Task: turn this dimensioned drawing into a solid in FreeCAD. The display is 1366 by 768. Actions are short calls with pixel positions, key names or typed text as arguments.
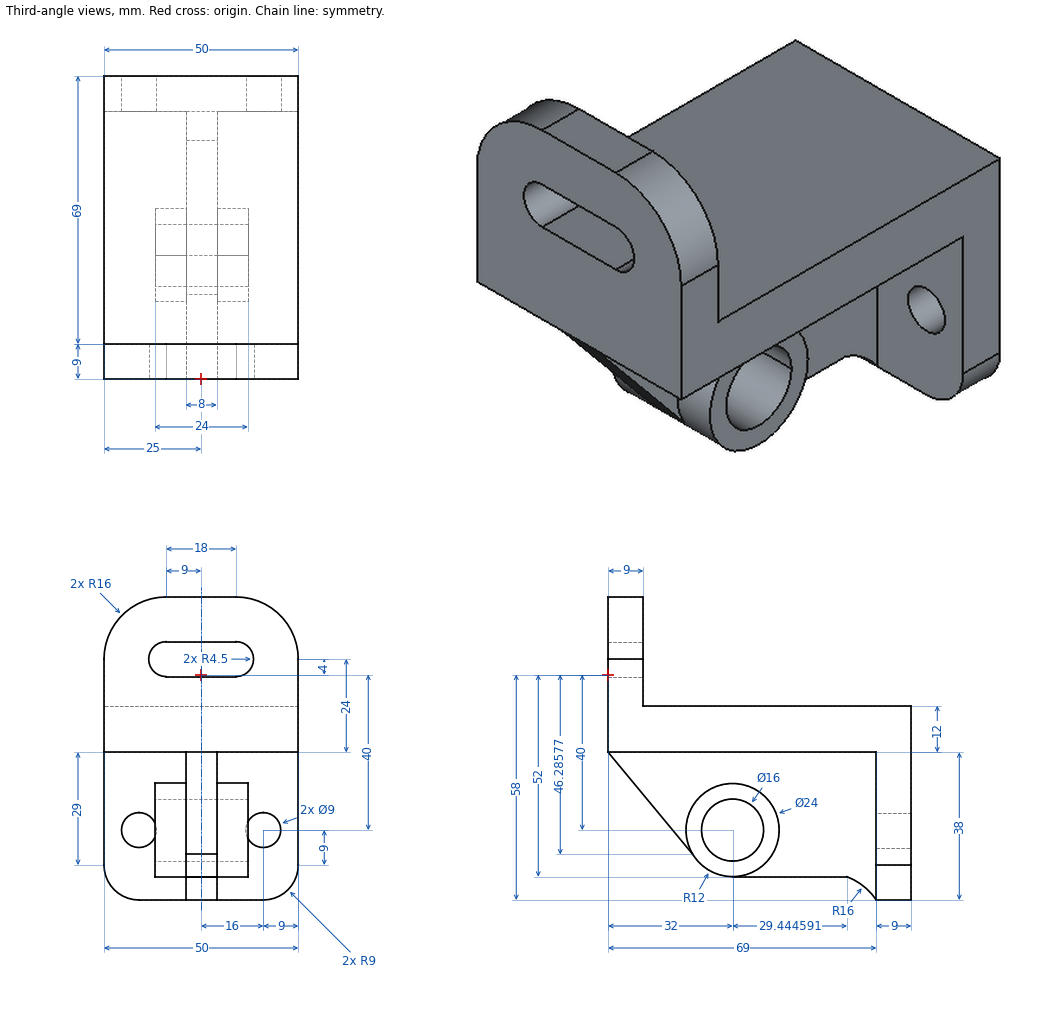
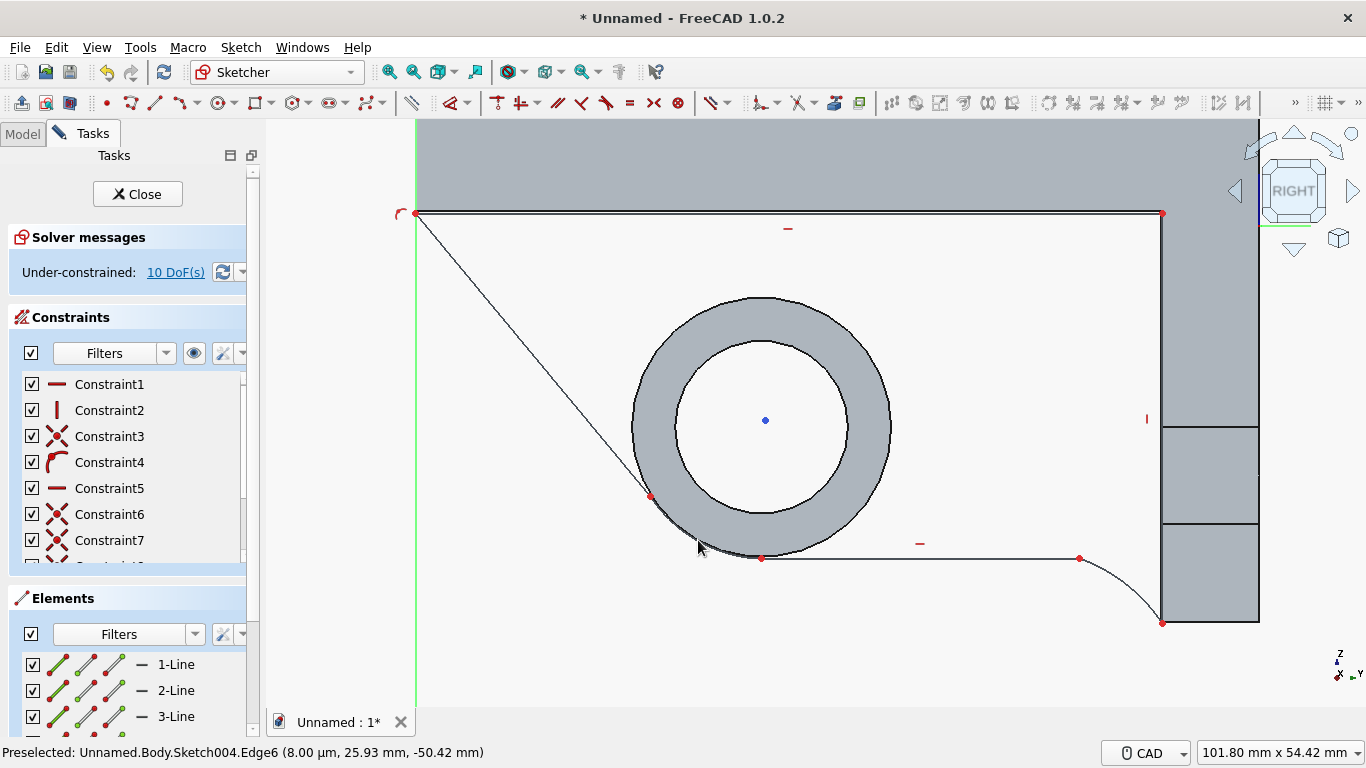
click(857, 559)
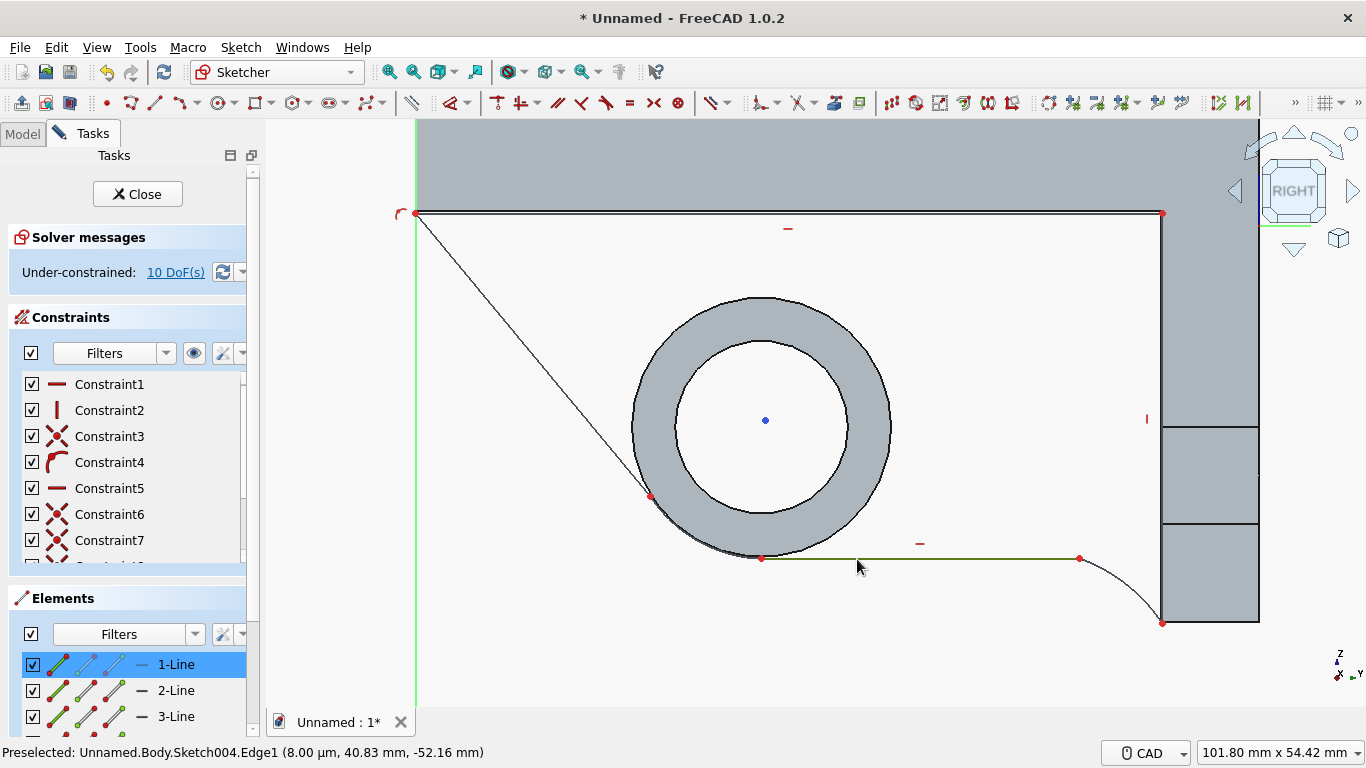
click(676, 526)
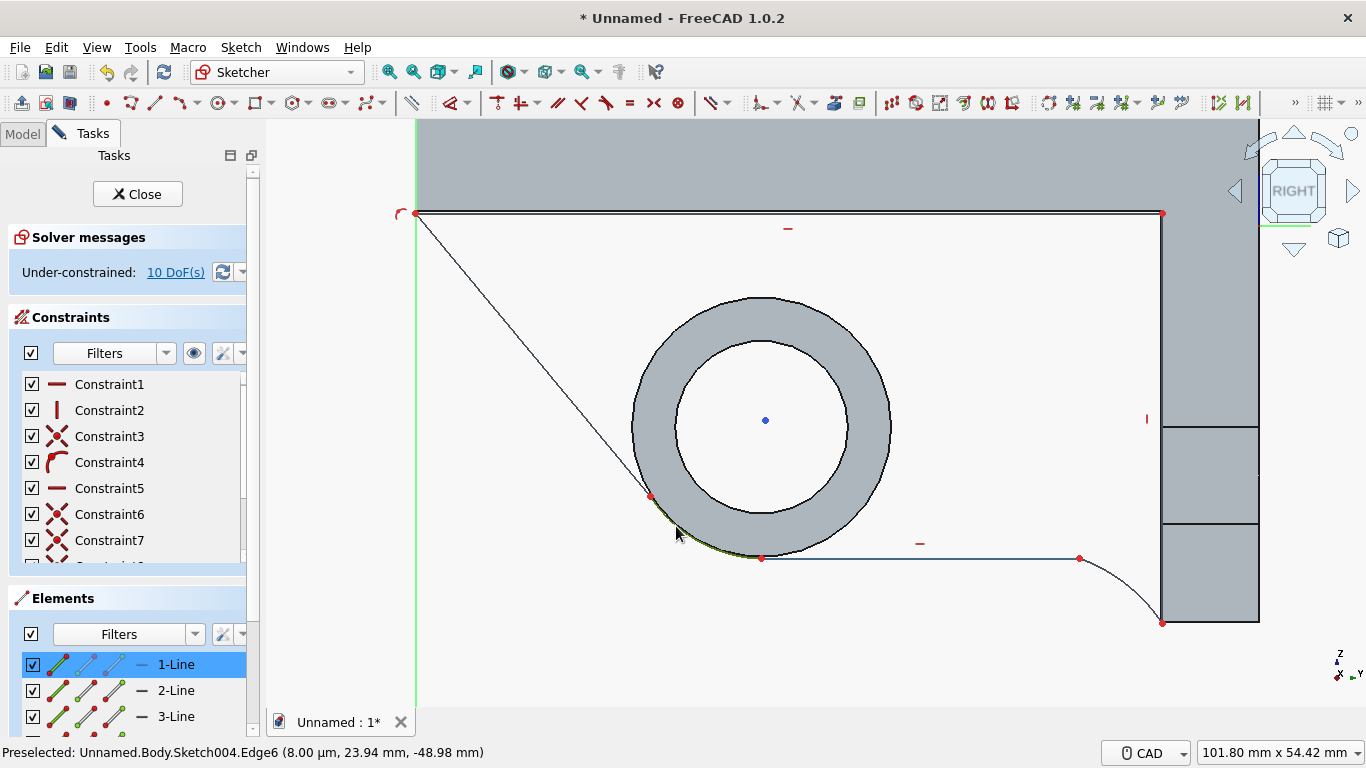
click(606, 104)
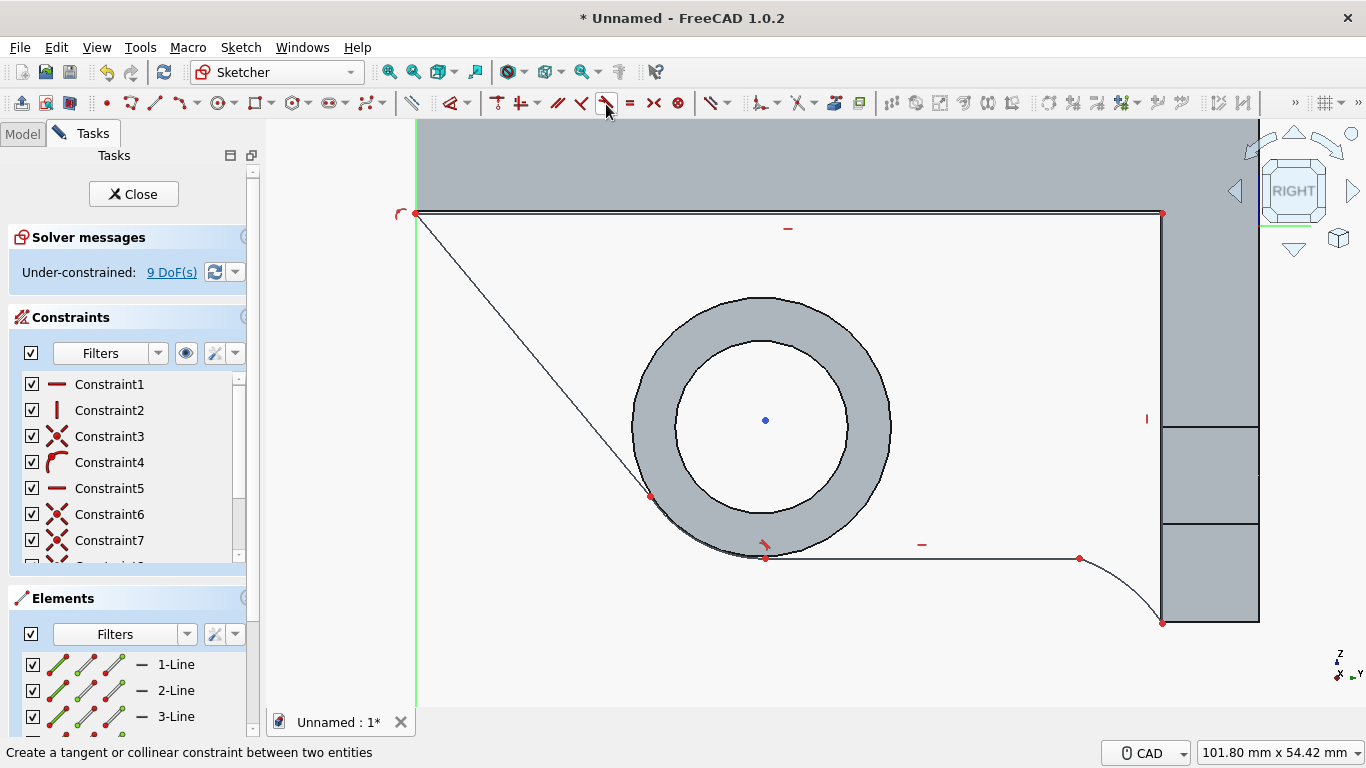
click(450, 104)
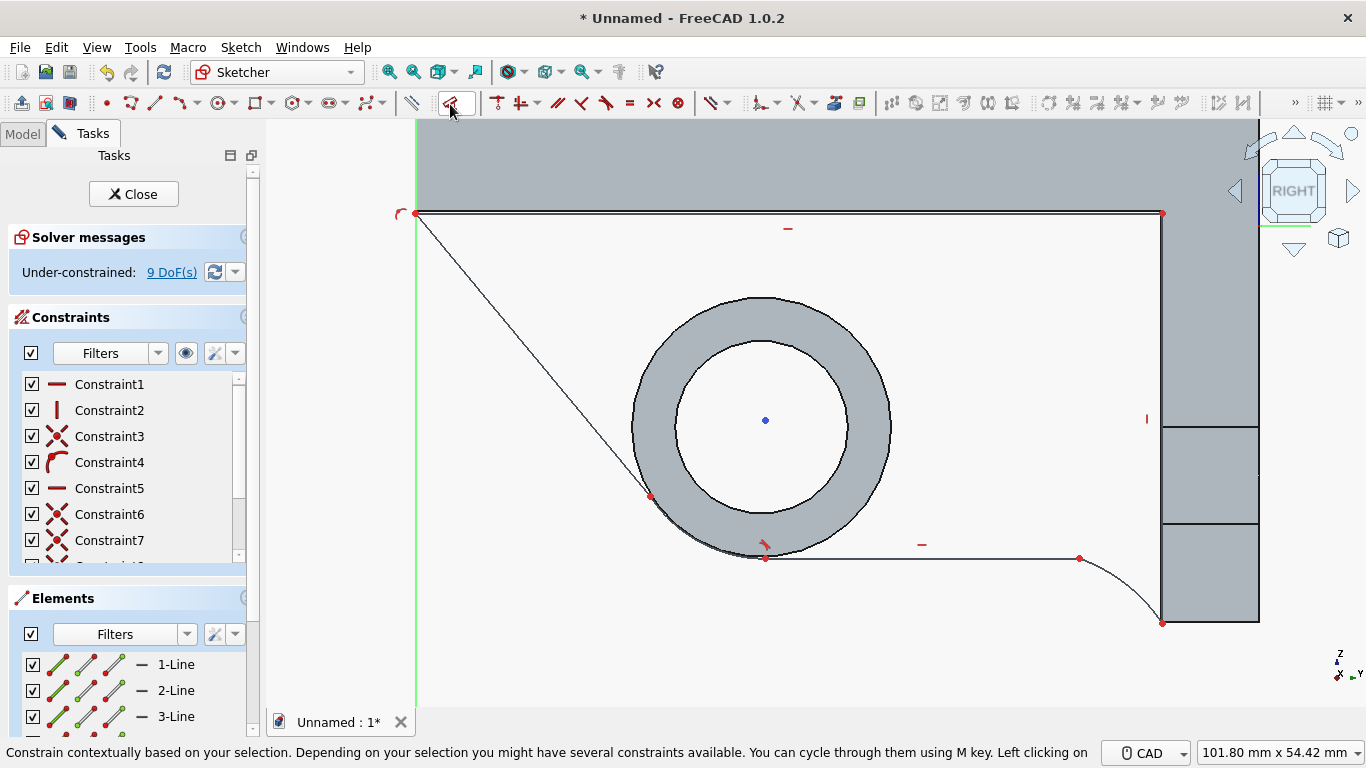
click(1142, 598)
click(1081, 525)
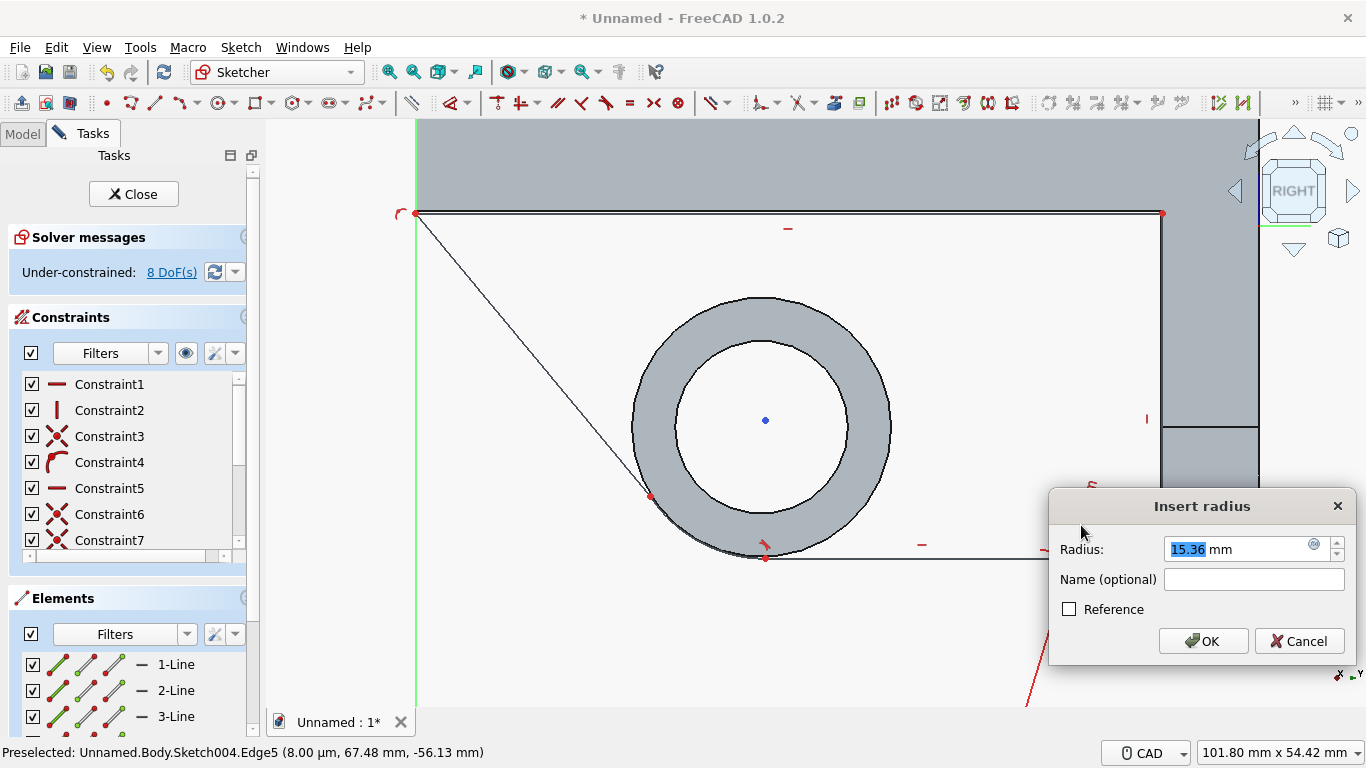
text(16)
key(Return)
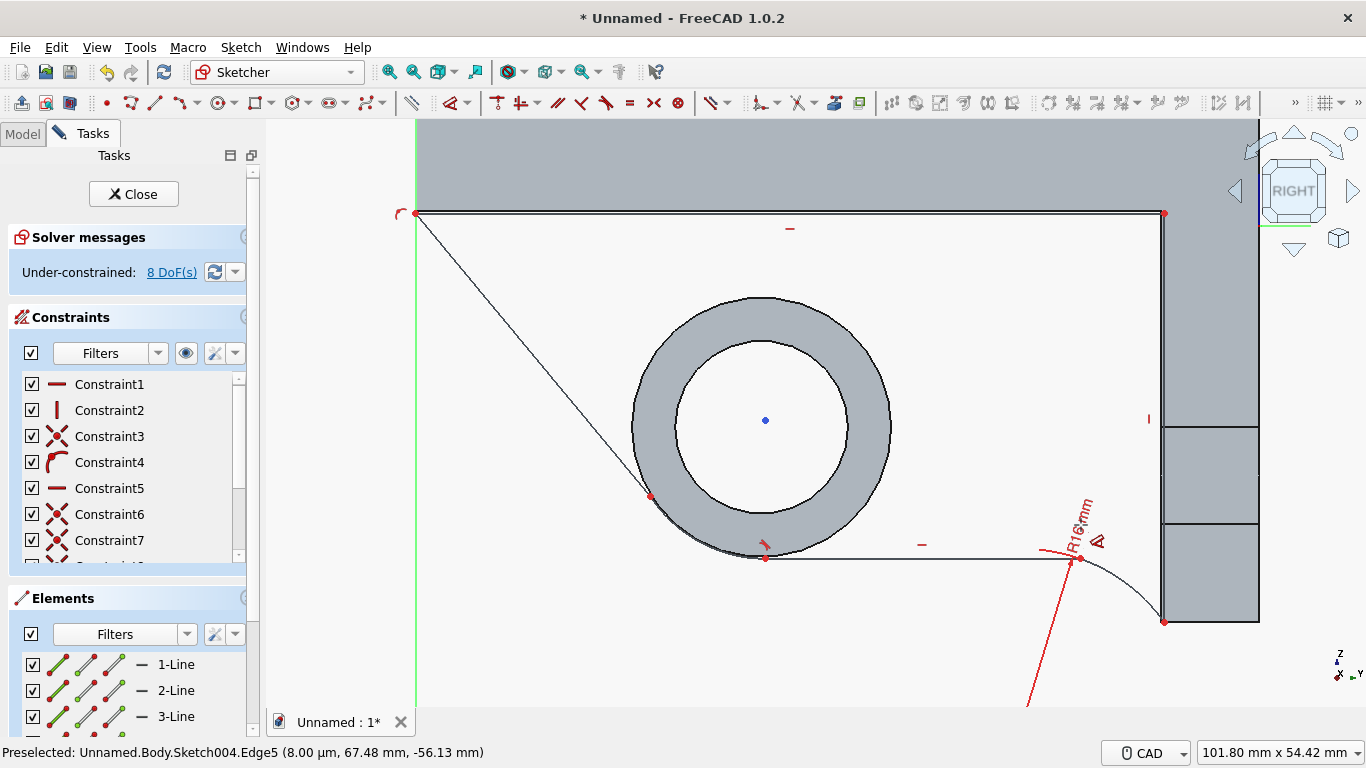
click(677, 527)
click(656, 552)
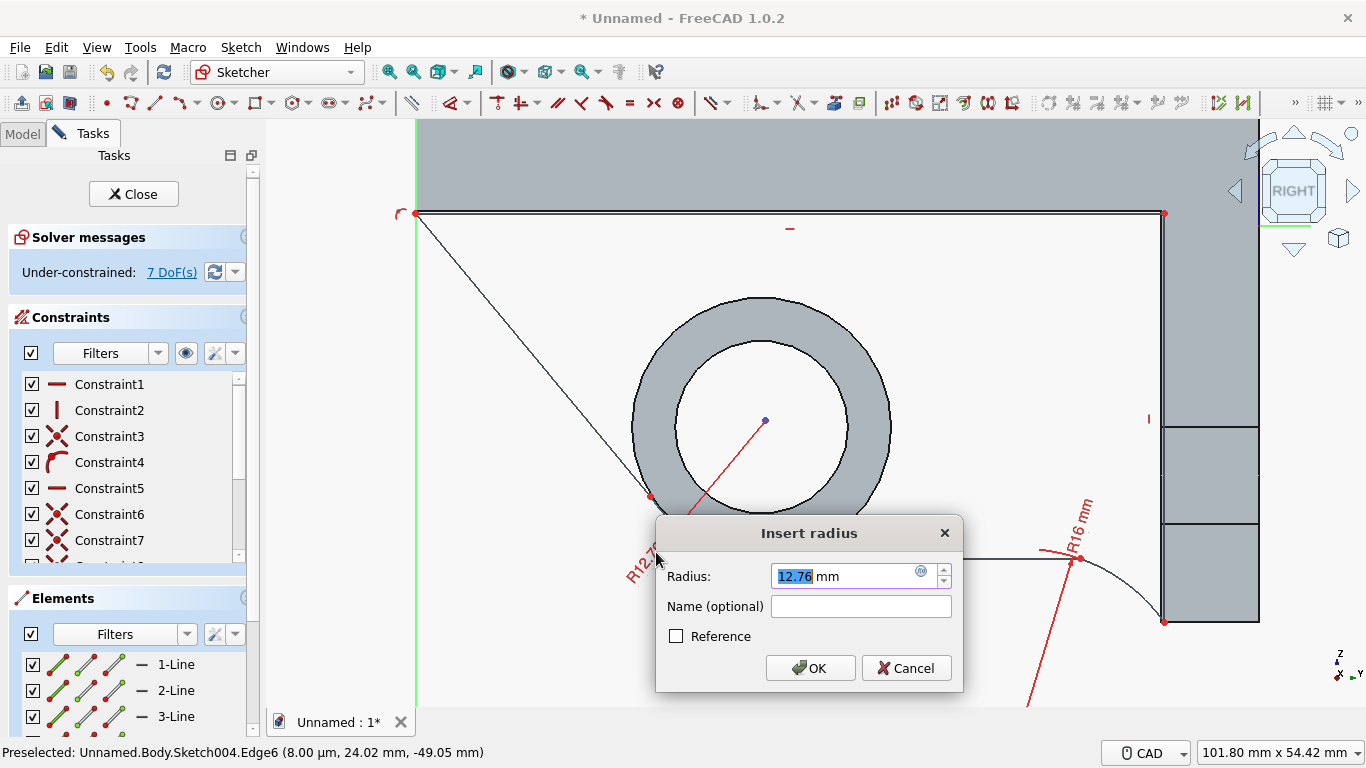
text(12)
key(Return)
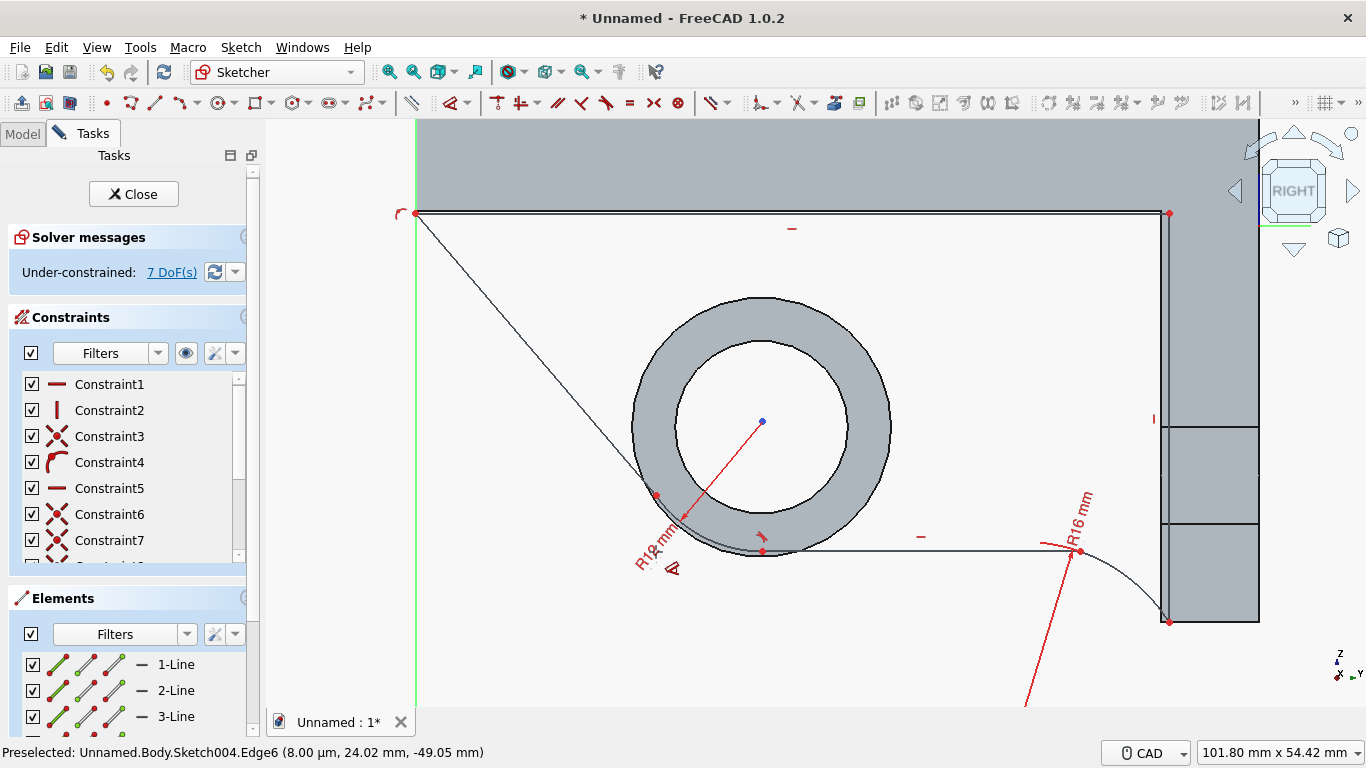
click(1169, 500)
click(1135, 418)